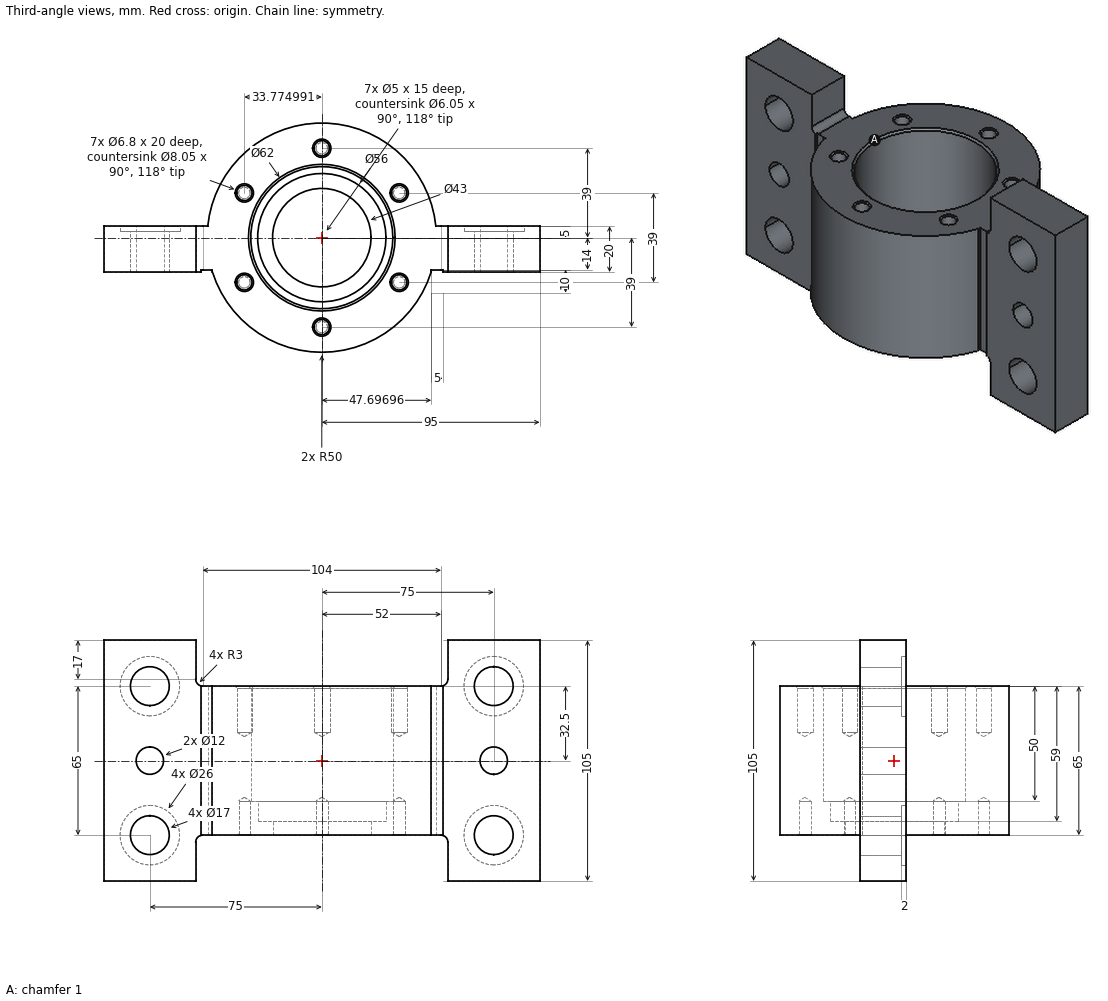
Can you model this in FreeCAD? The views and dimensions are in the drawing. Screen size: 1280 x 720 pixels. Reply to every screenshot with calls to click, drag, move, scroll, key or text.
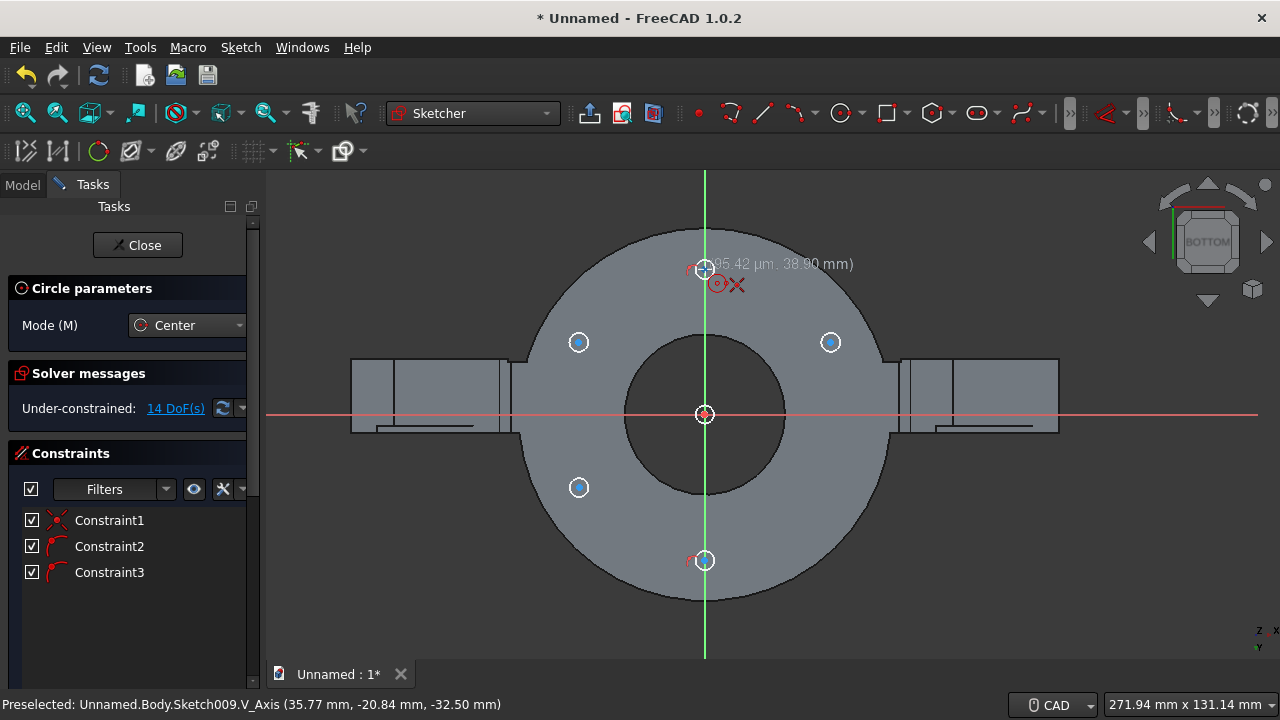
scroll(831, 487, up, 5)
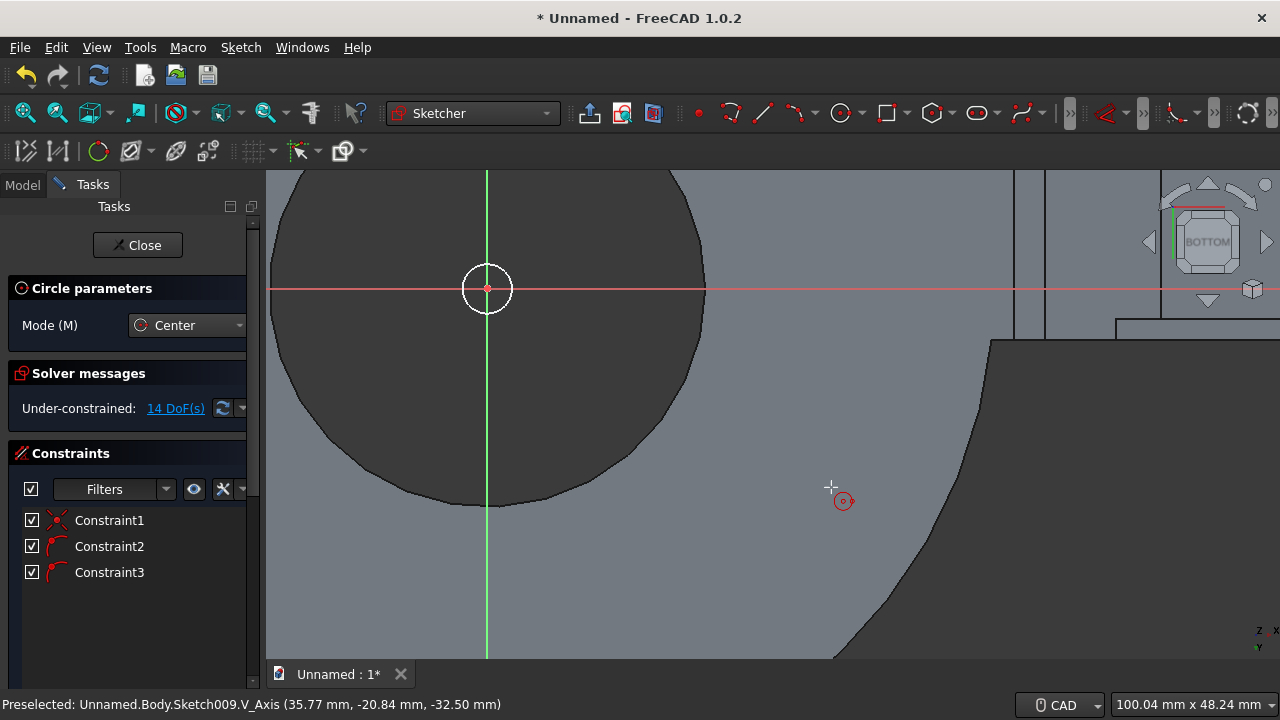
click(830, 487)
click(848, 469)
key(Escape)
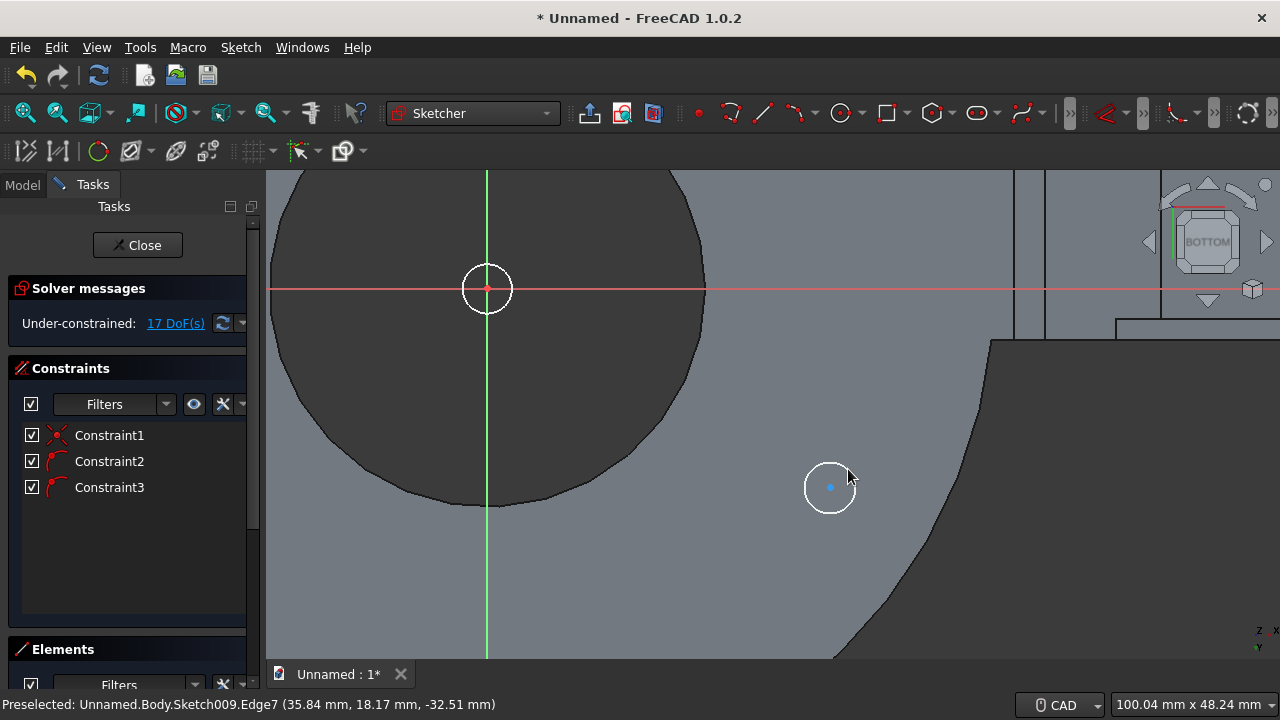
click(505, 271)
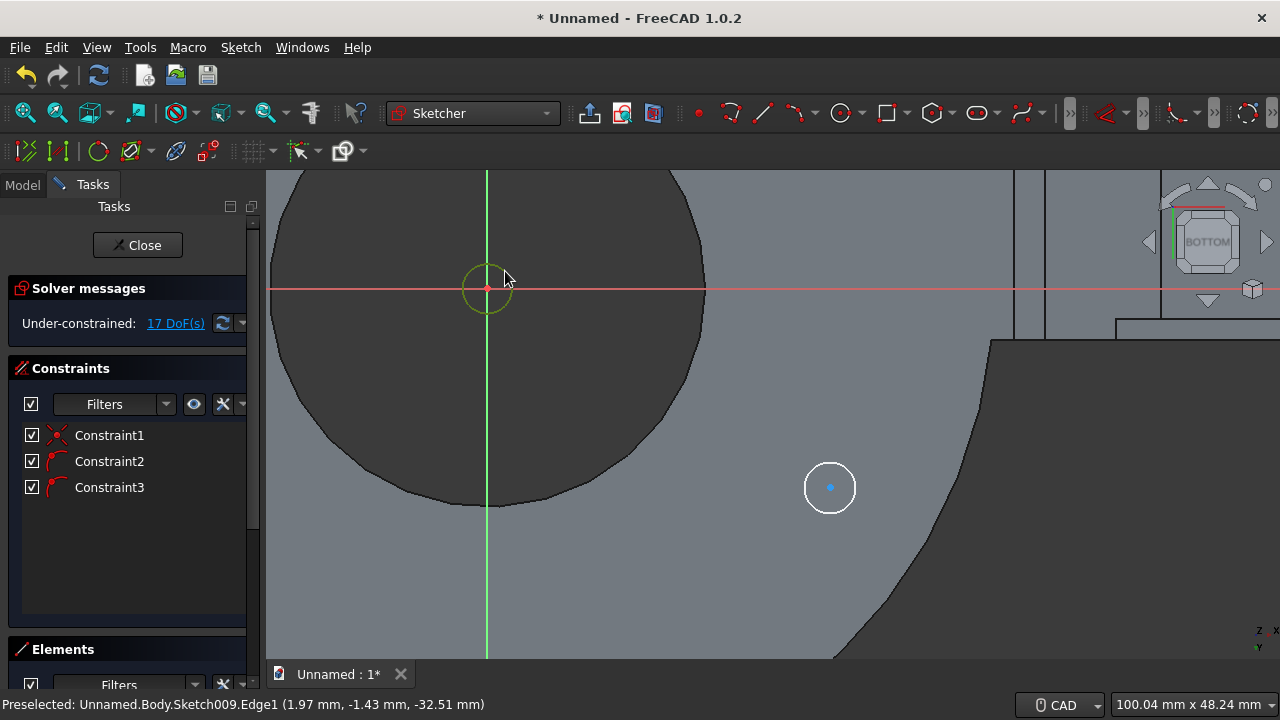
scroll(831, 488, down, 5)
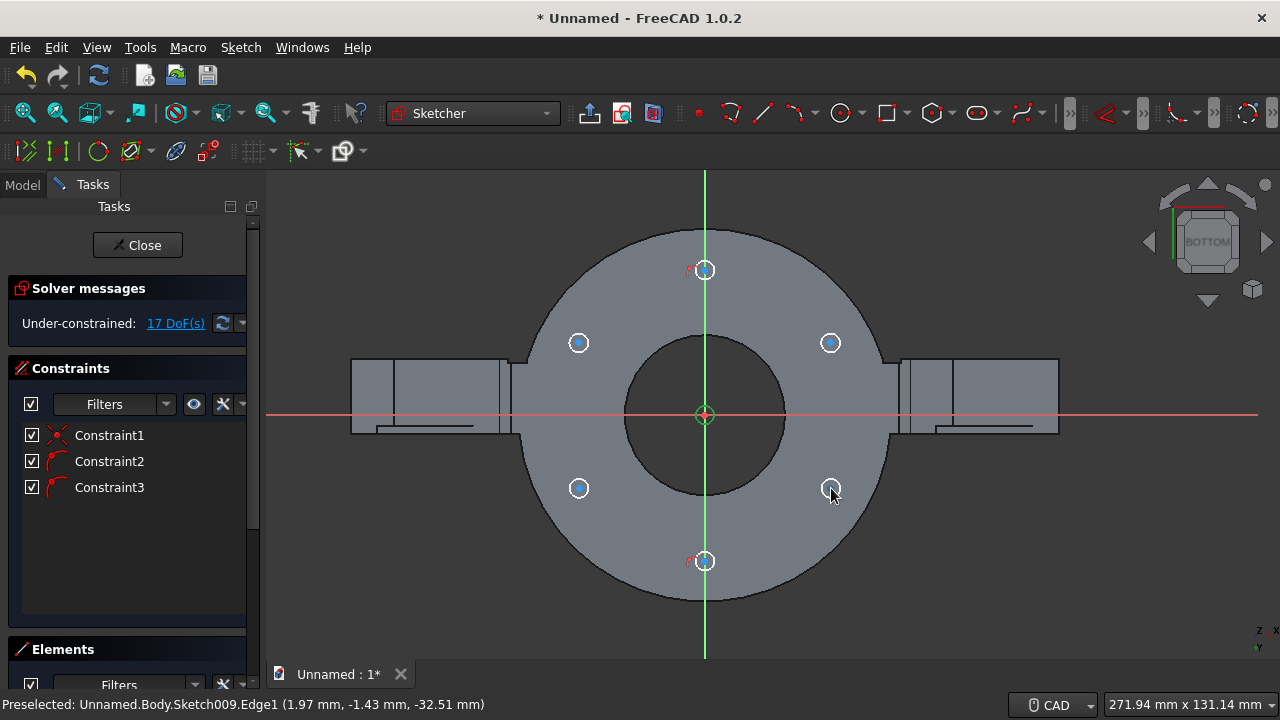
scroll(712, 555, up, 4)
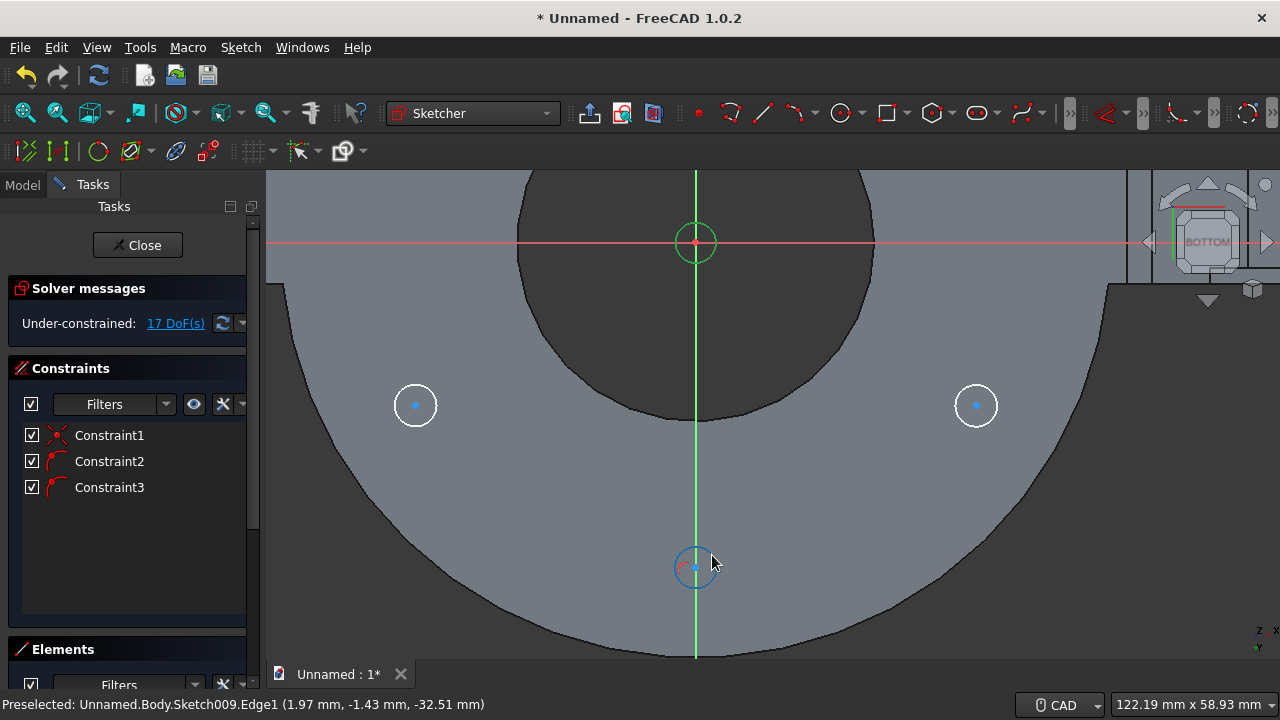
click(710, 553)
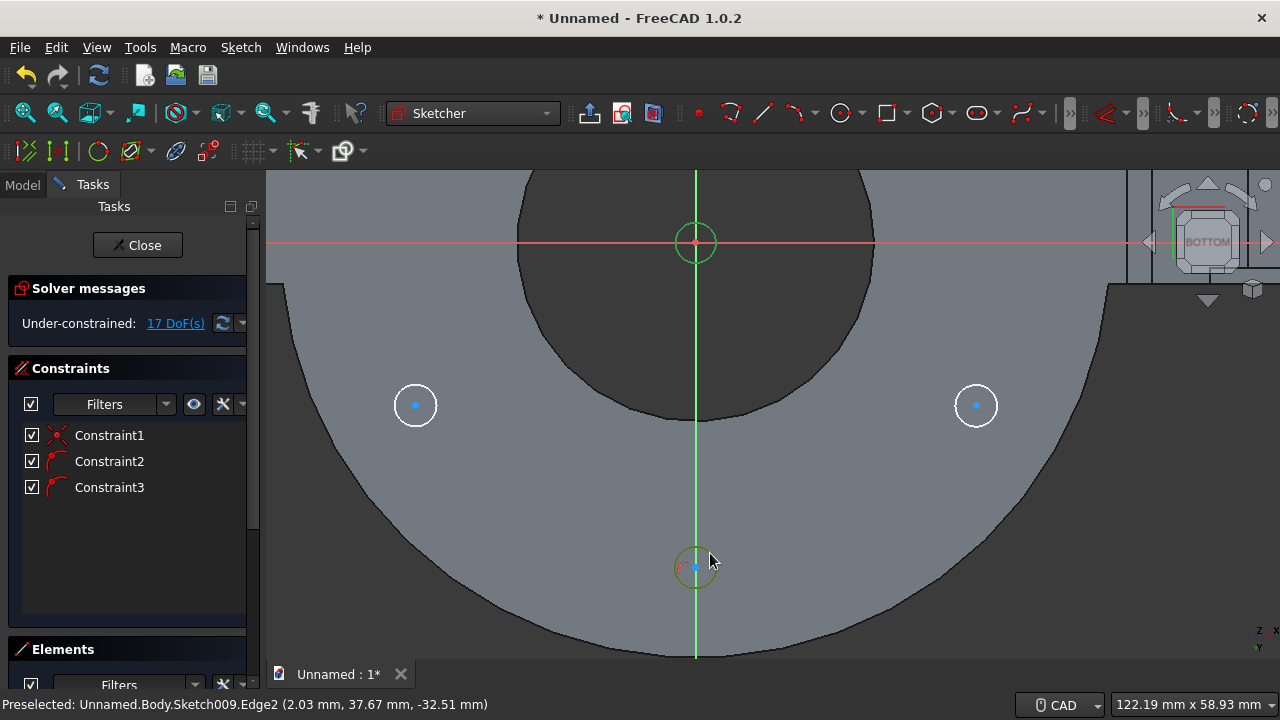
click(430, 391)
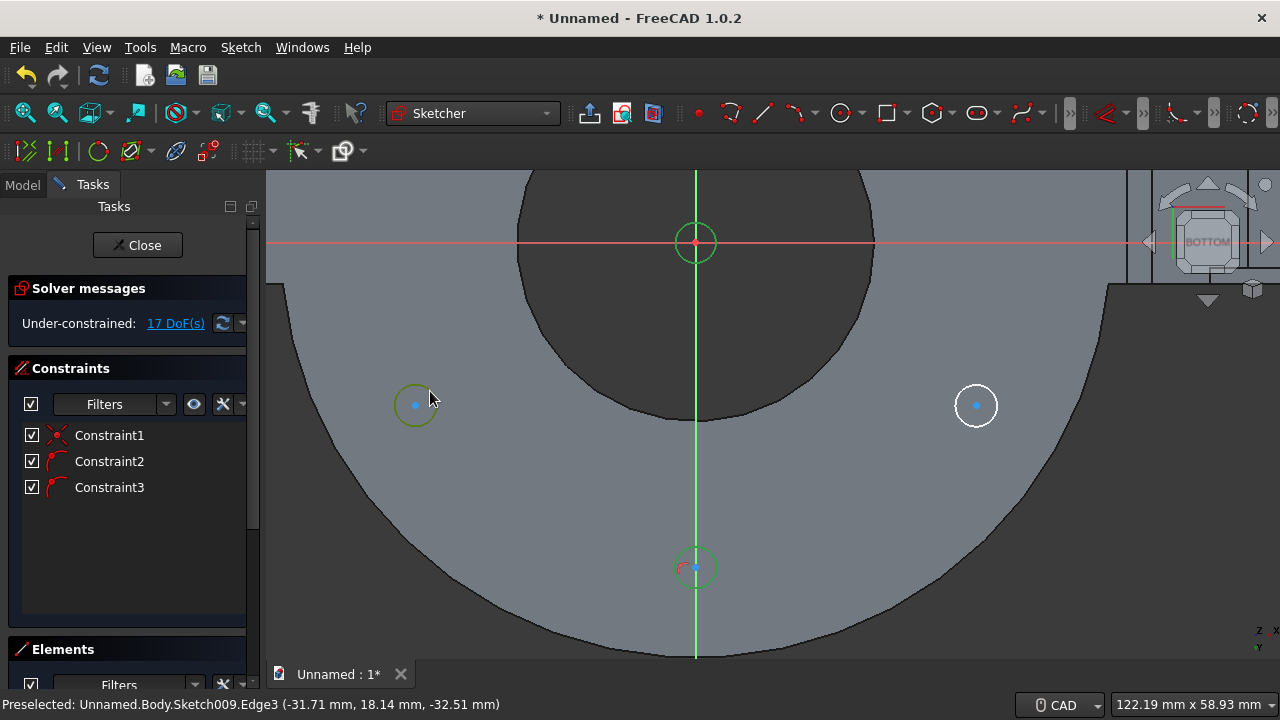
scroll(712, 555, down, 4)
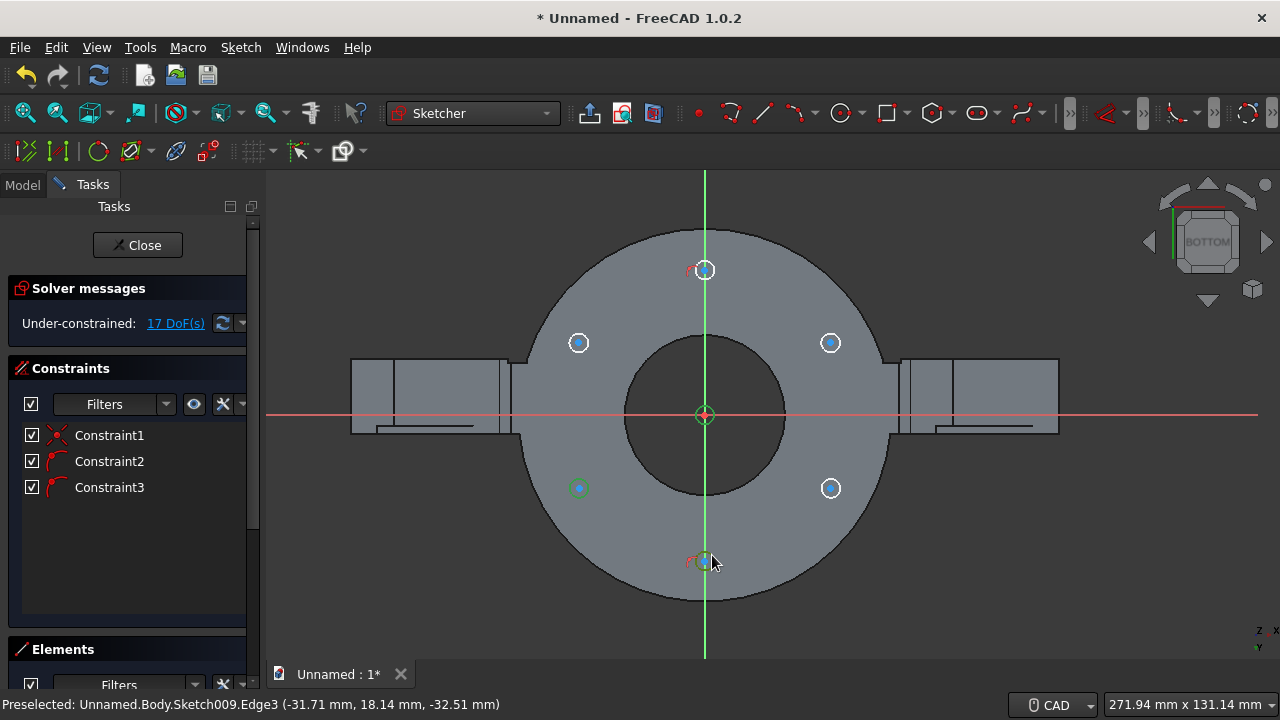
scroll(585, 336, up, 2)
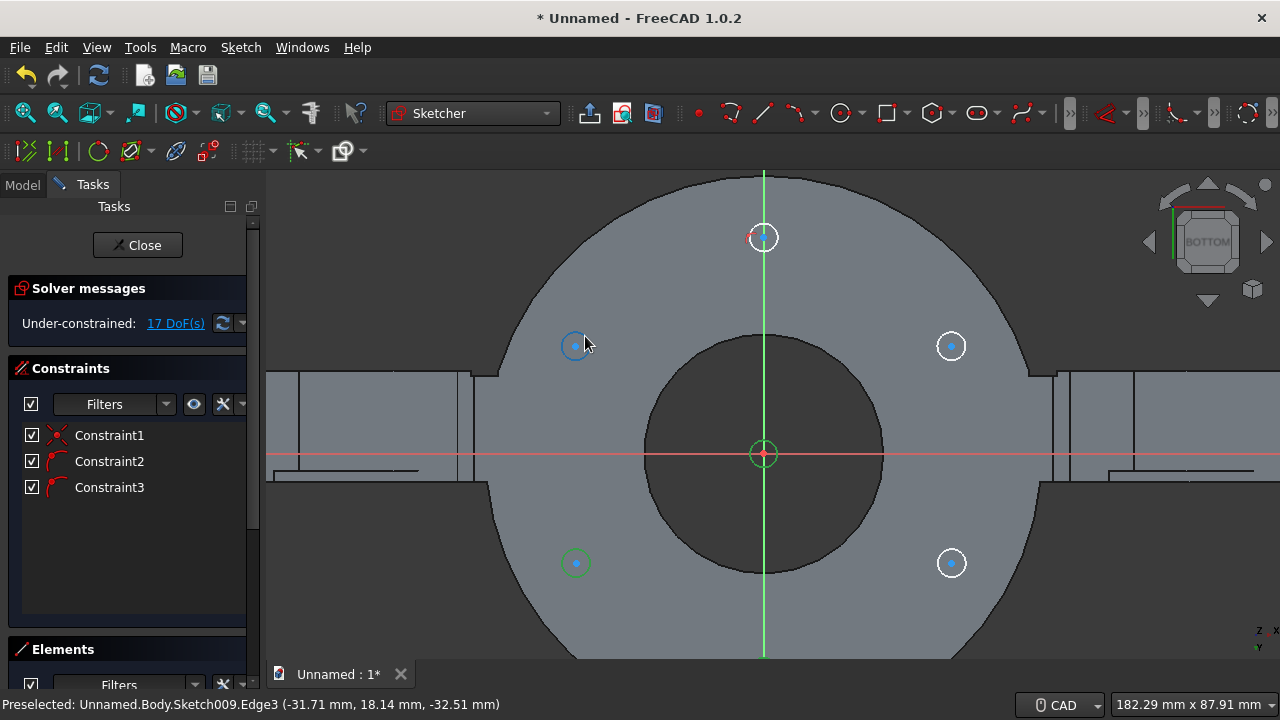
click(585, 336)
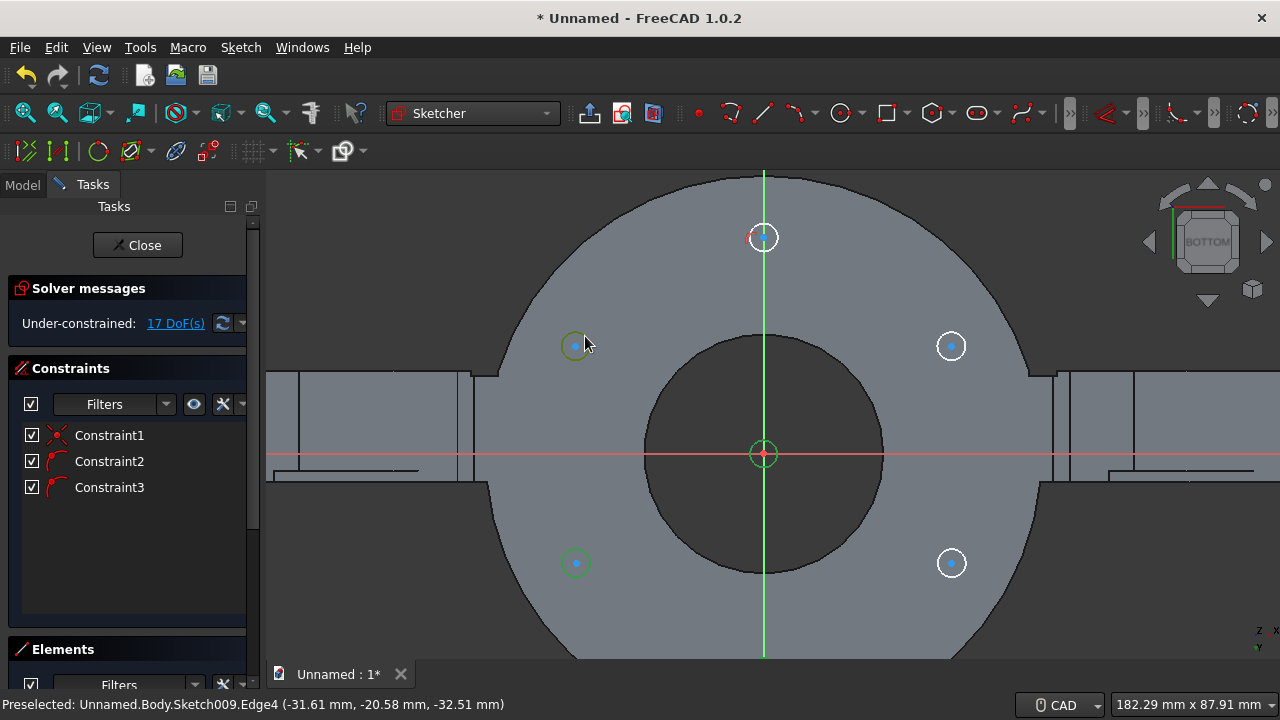
scroll(774, 228, up, 2)